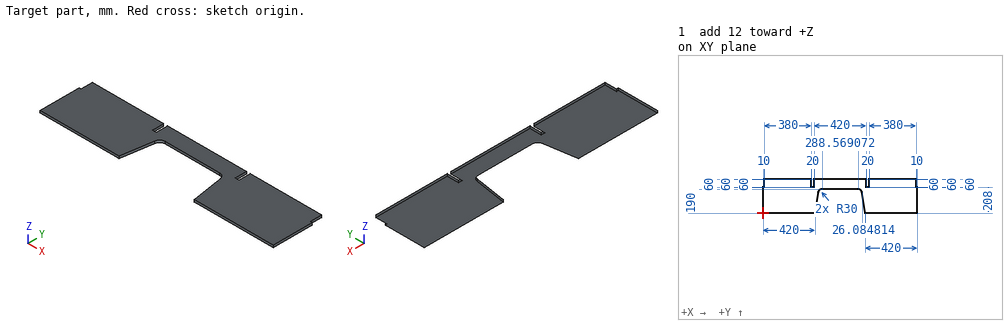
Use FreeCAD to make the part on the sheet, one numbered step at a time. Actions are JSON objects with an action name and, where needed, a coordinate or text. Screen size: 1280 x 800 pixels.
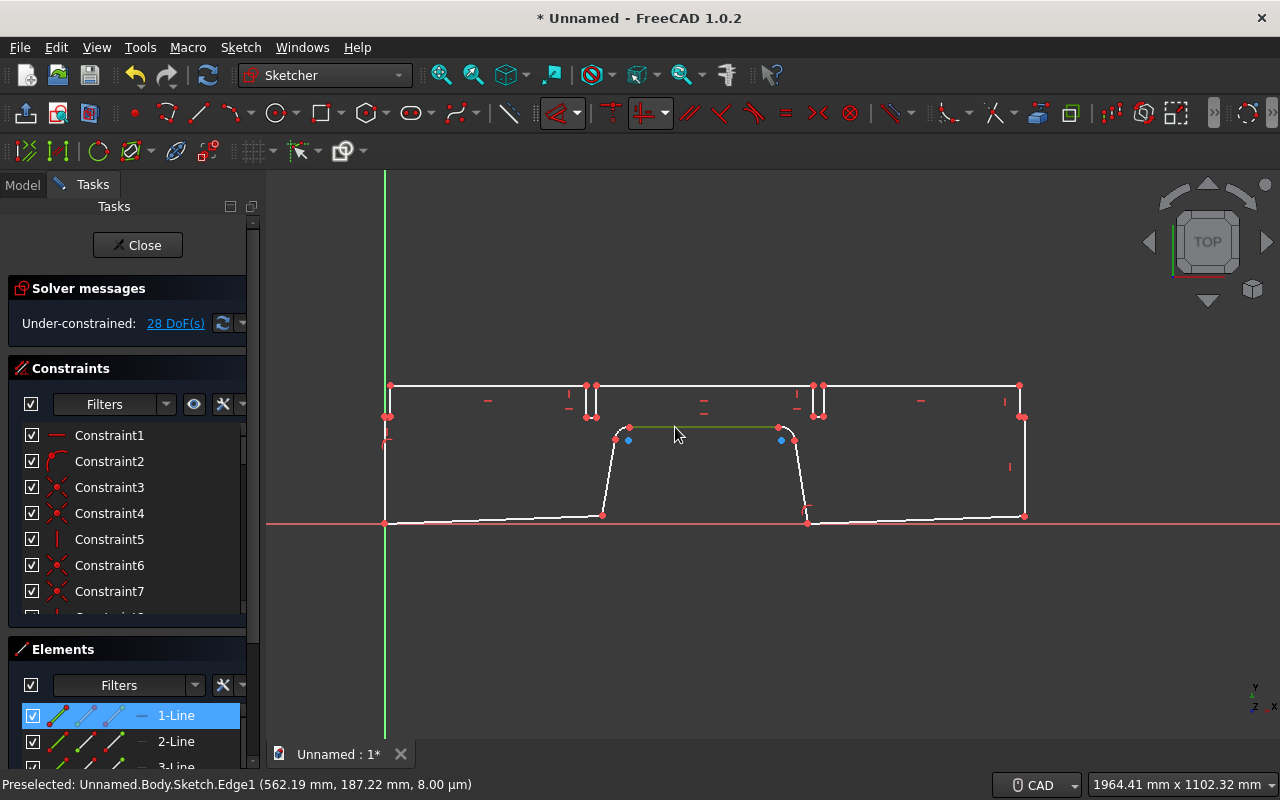
{"action": "left_click", "coordinate": [790, 430]}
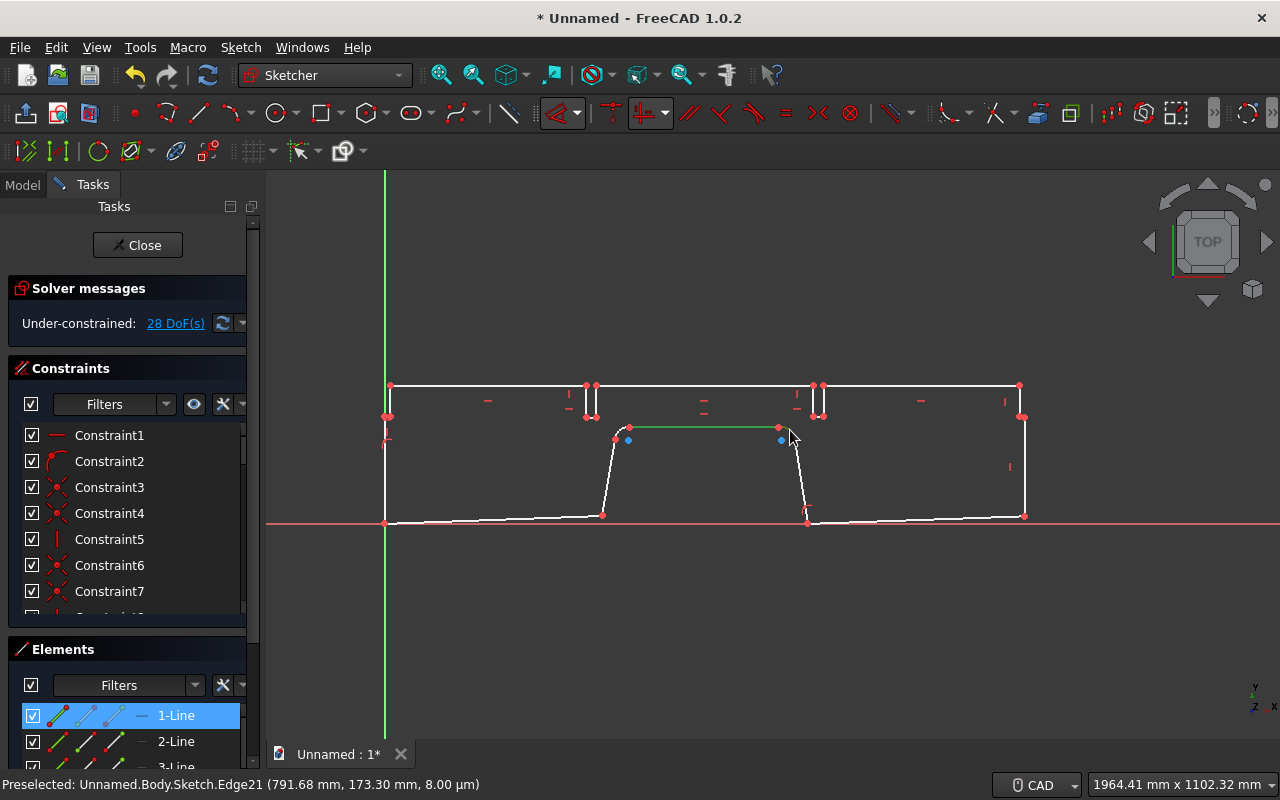
{"action": "left_click", "coordinate": [754, 114]}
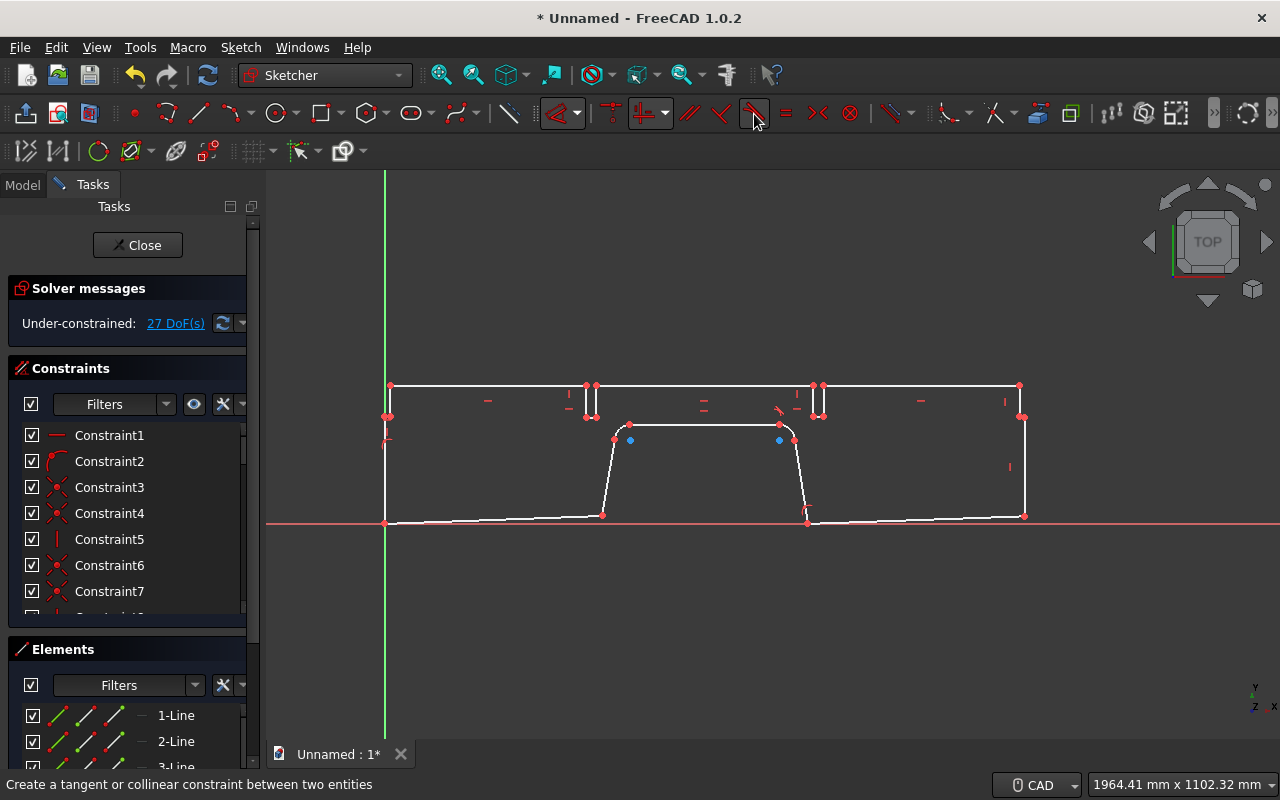
{"action": "left_click", "coordinate": [675, 425]}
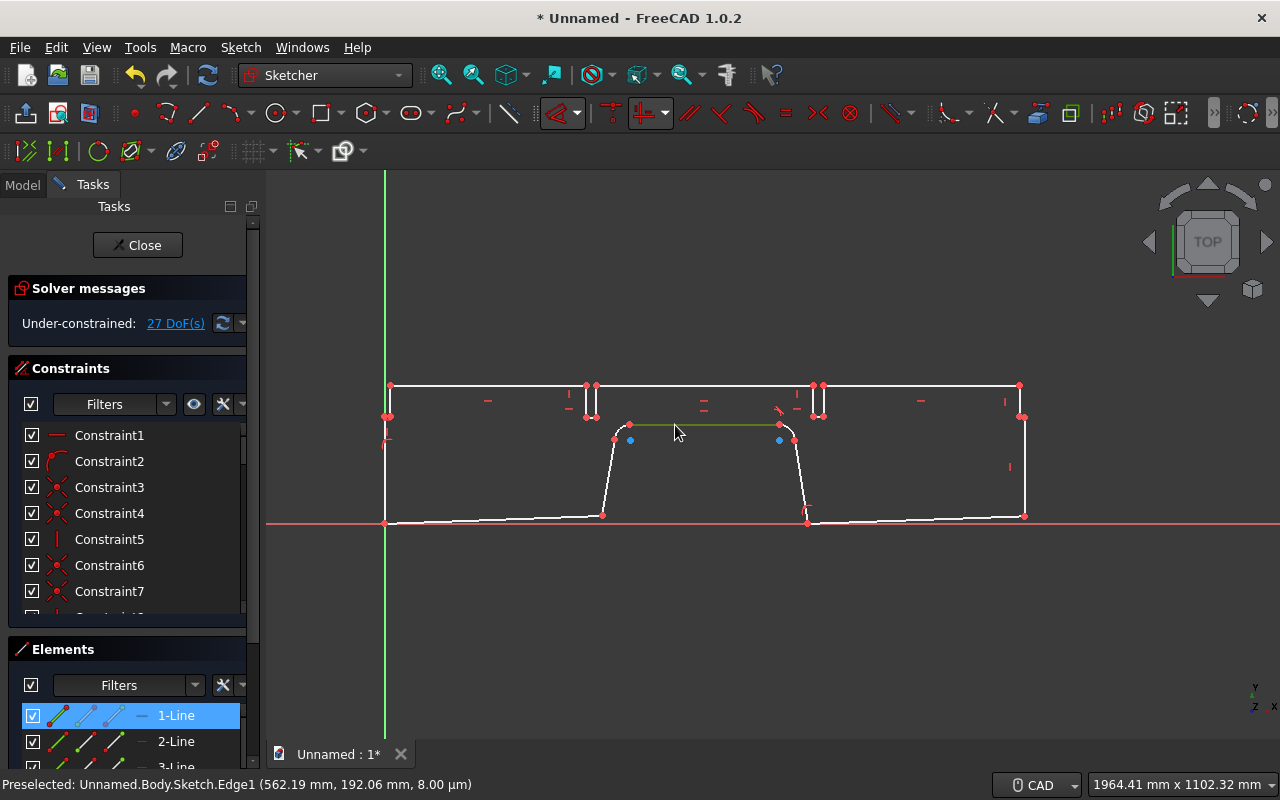
{"action": "left_click", "coordinate": [619, 429]}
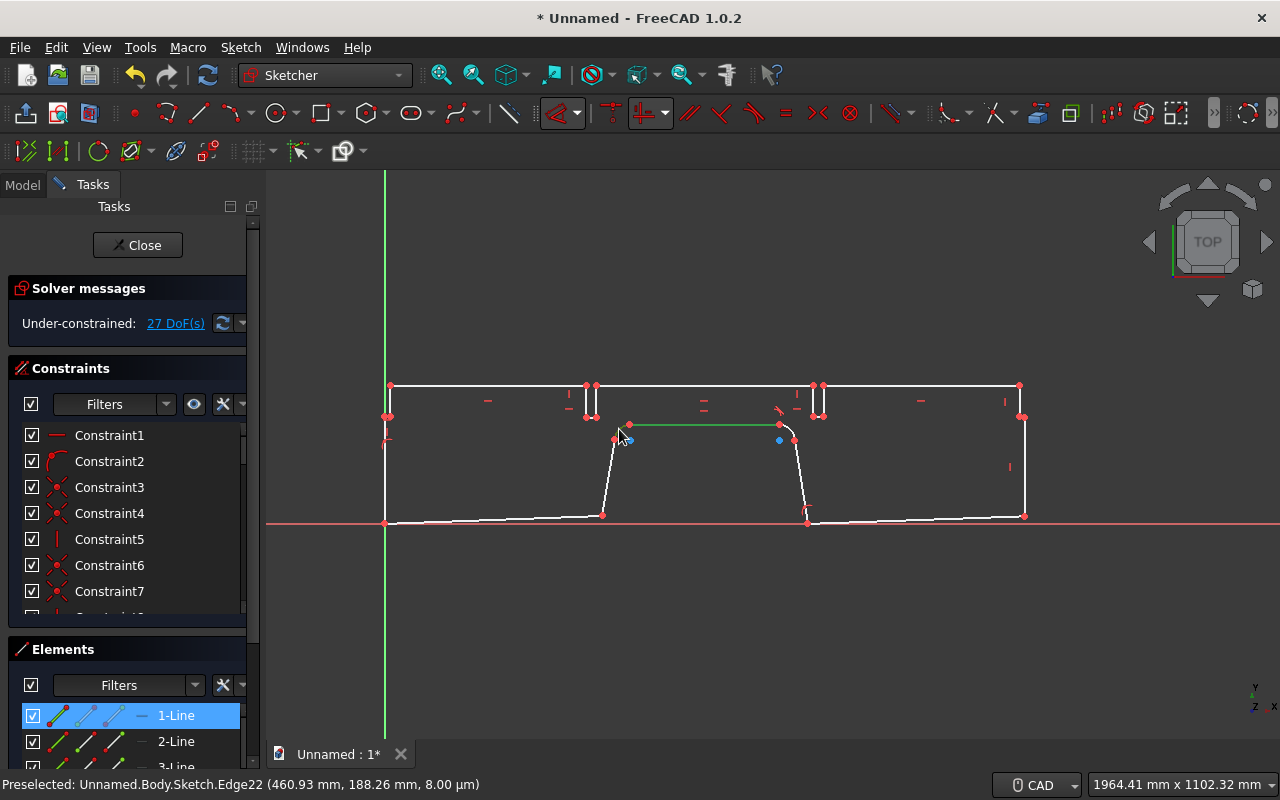
{"action": "key", "text": "t"}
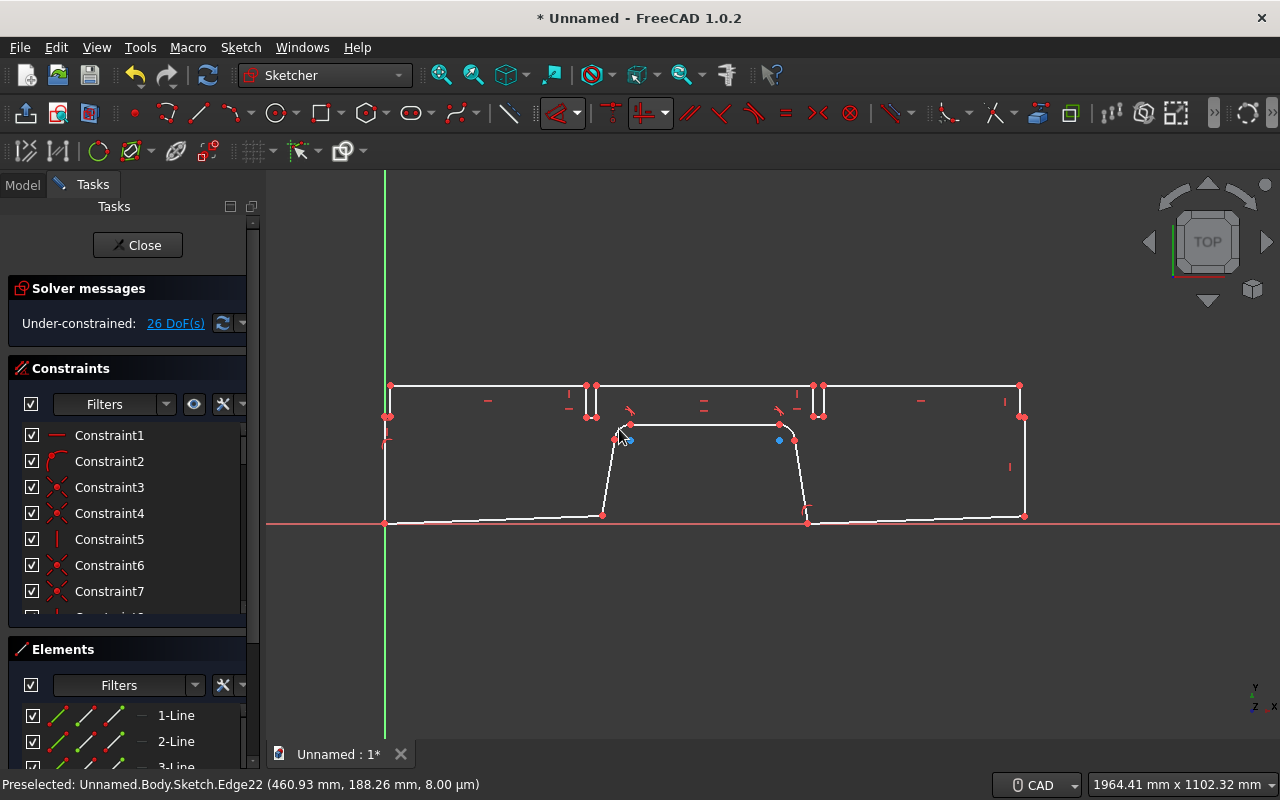
{"action": "left_click", "coordinate": [799, 465]}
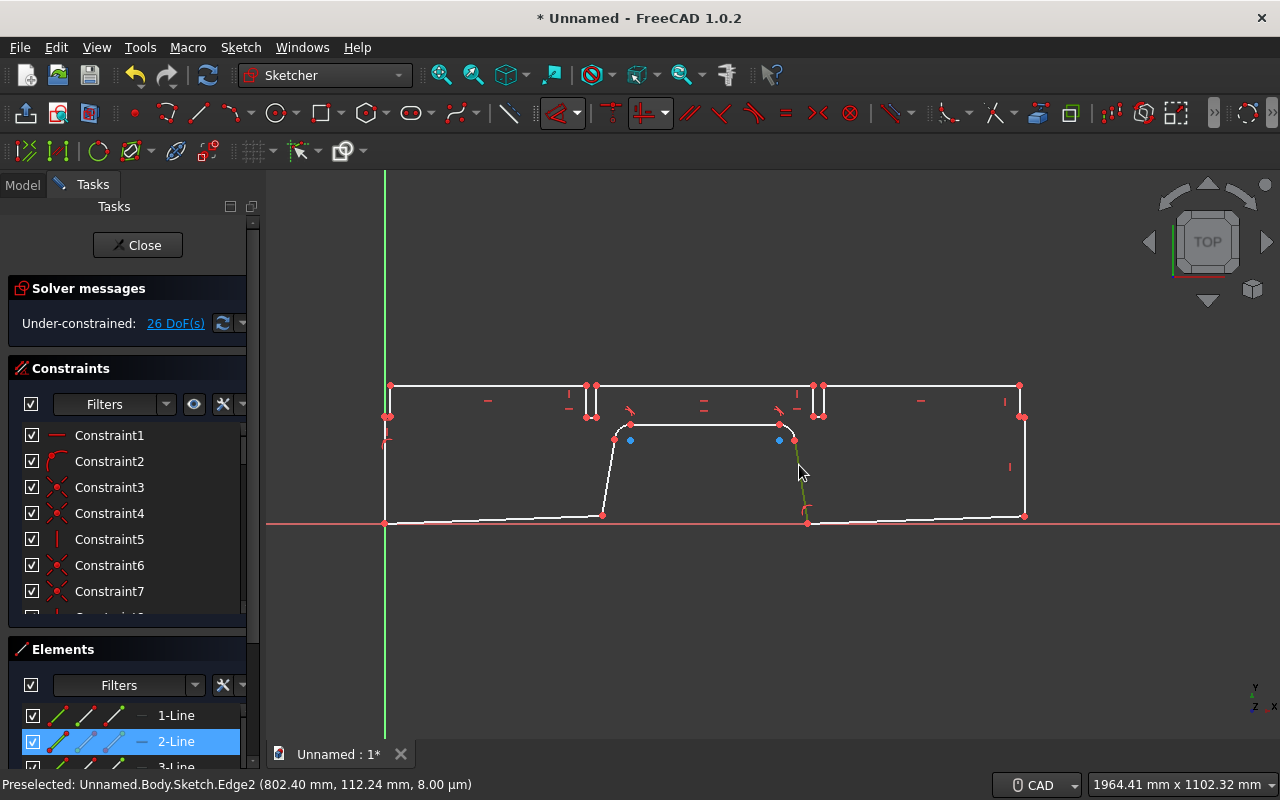
{"action": "left_click", "coordinate": [790, 429]}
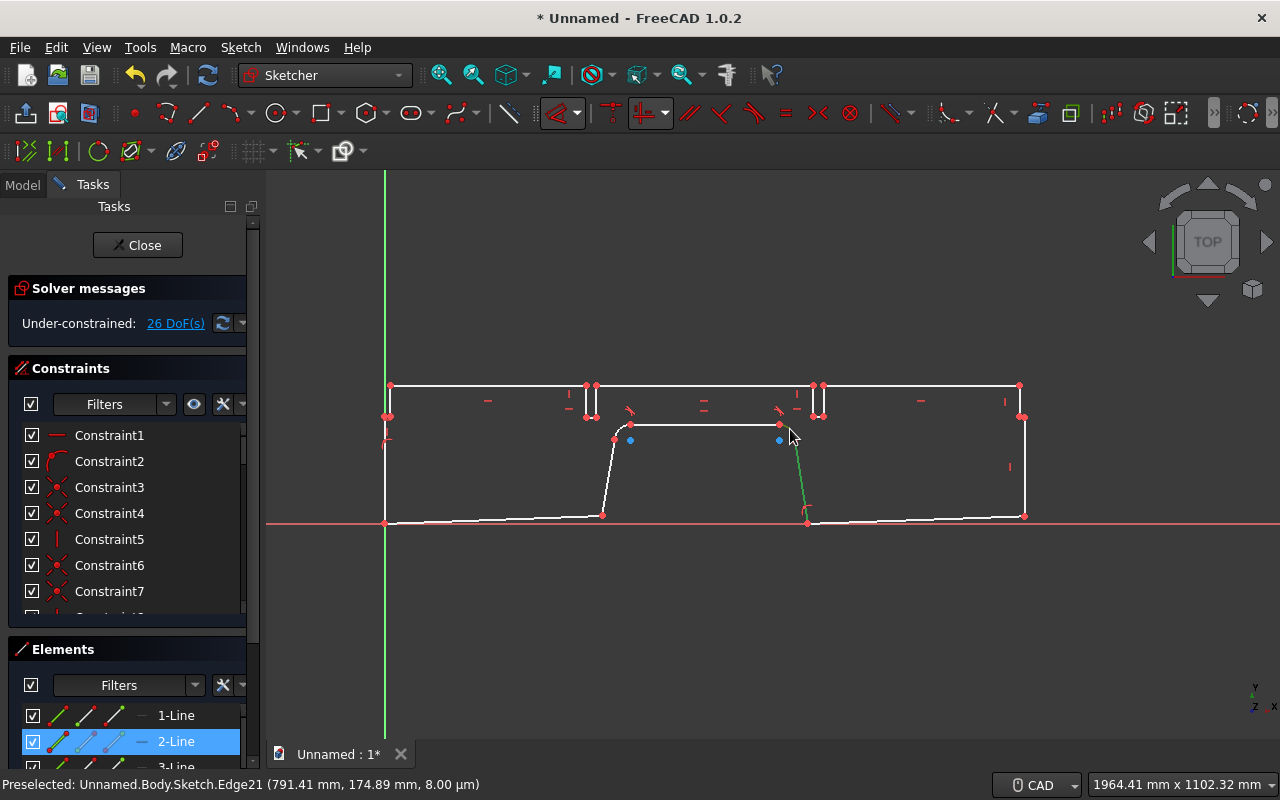
{"action": "key", "text": "t"}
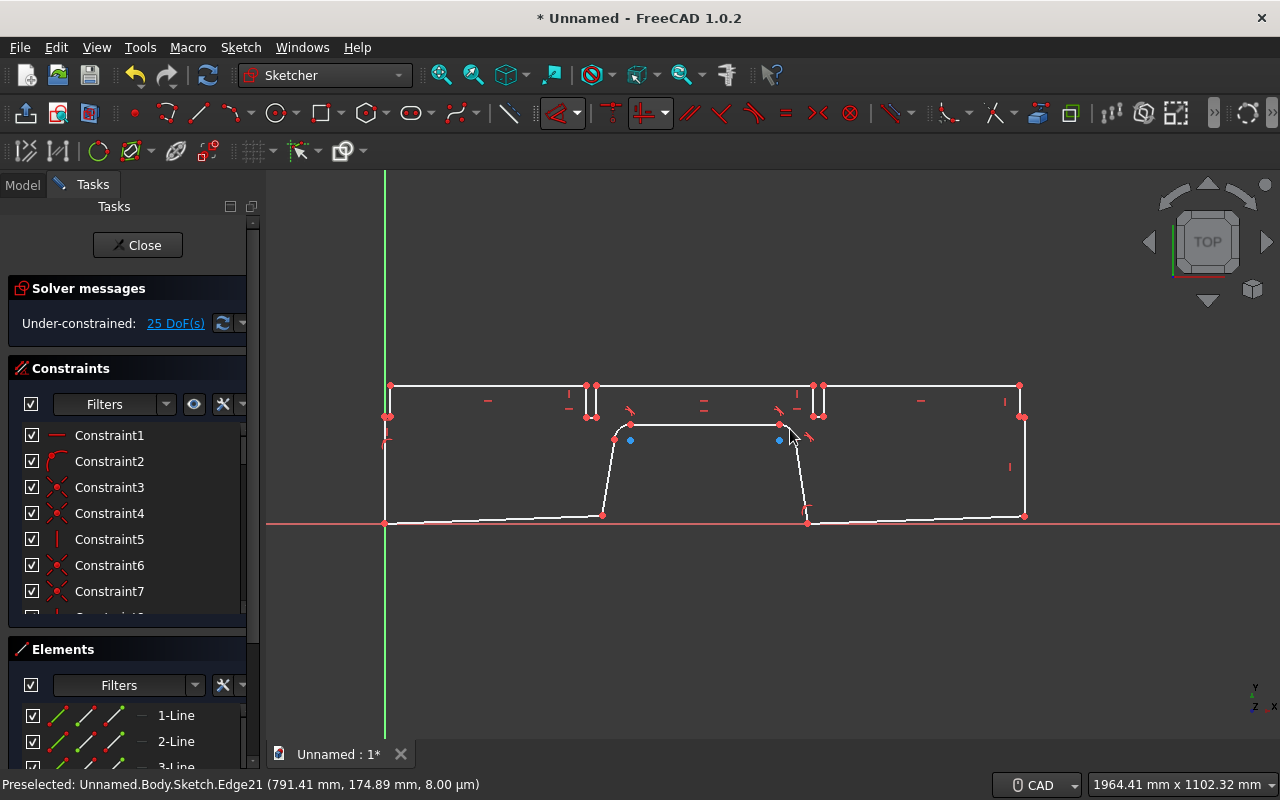
{"action": "left_click", "coordinate": [606, 493]}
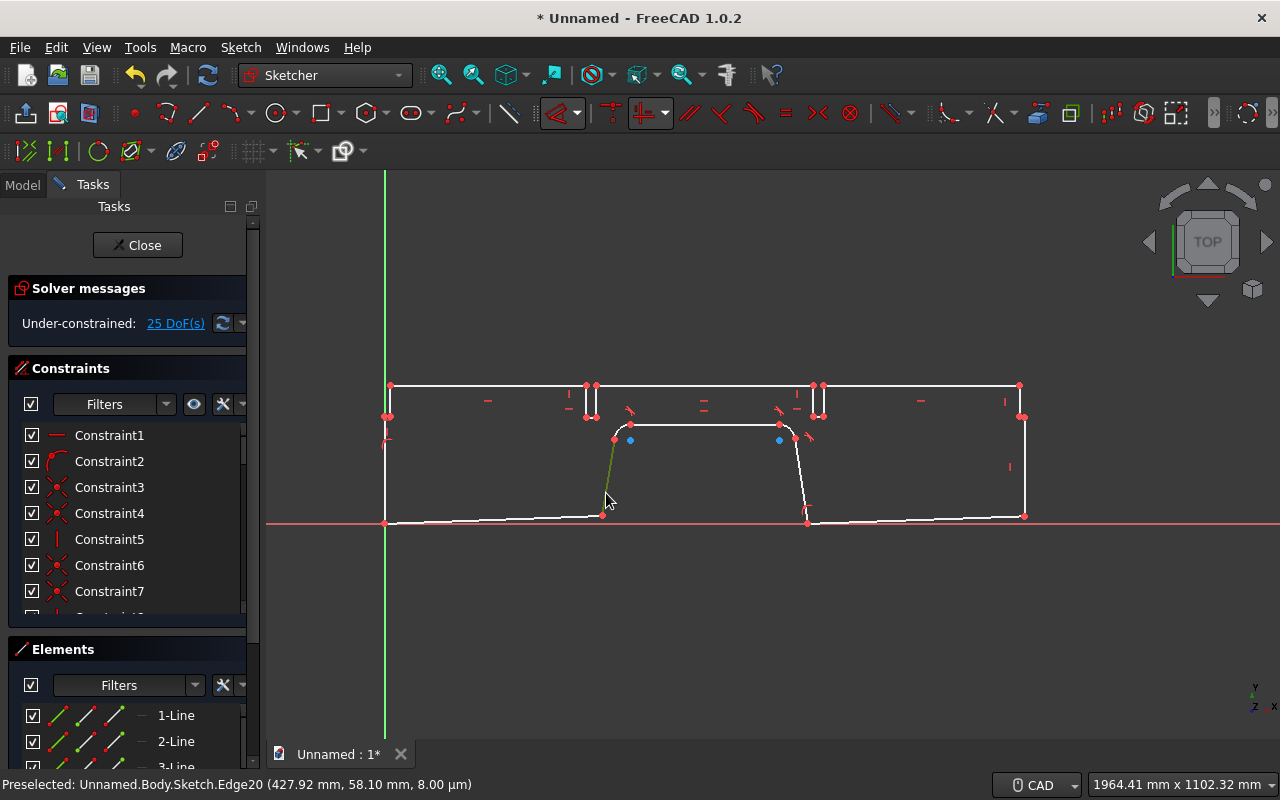
{"action": "left_click", "coordinate": [619, 429]}